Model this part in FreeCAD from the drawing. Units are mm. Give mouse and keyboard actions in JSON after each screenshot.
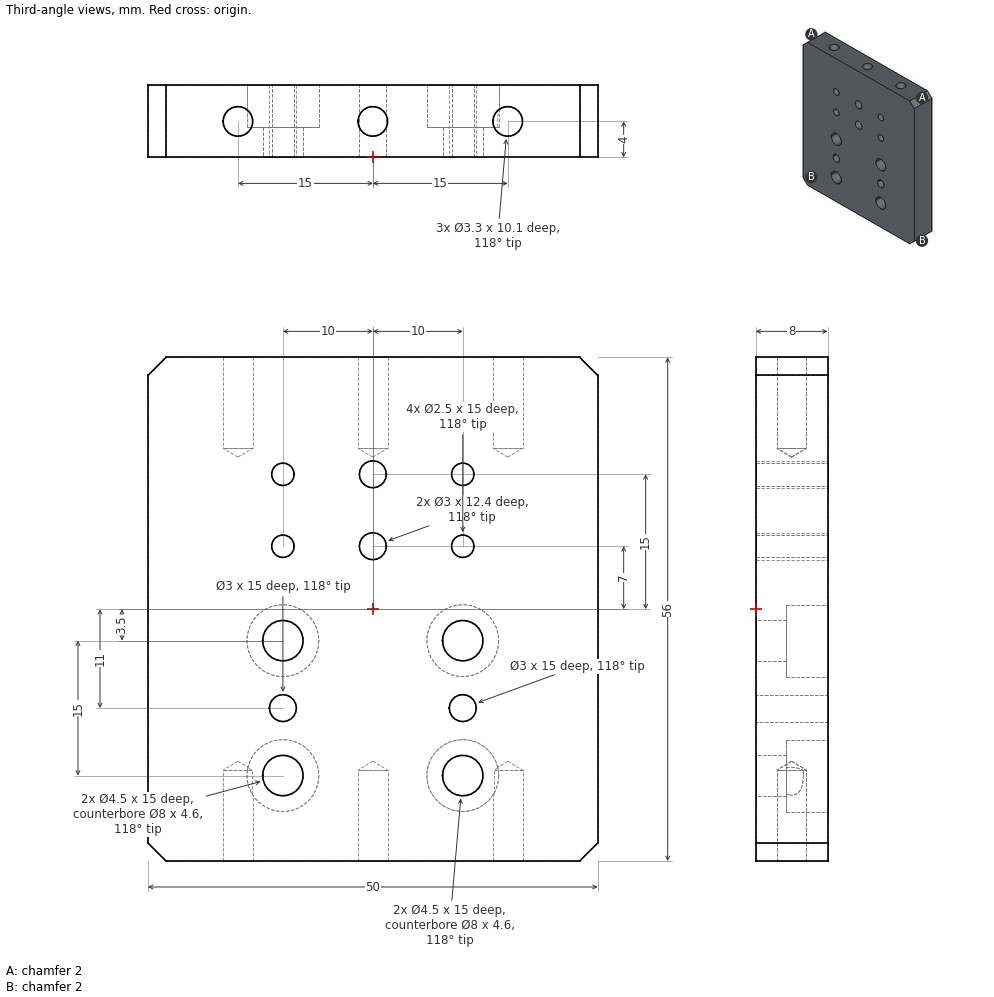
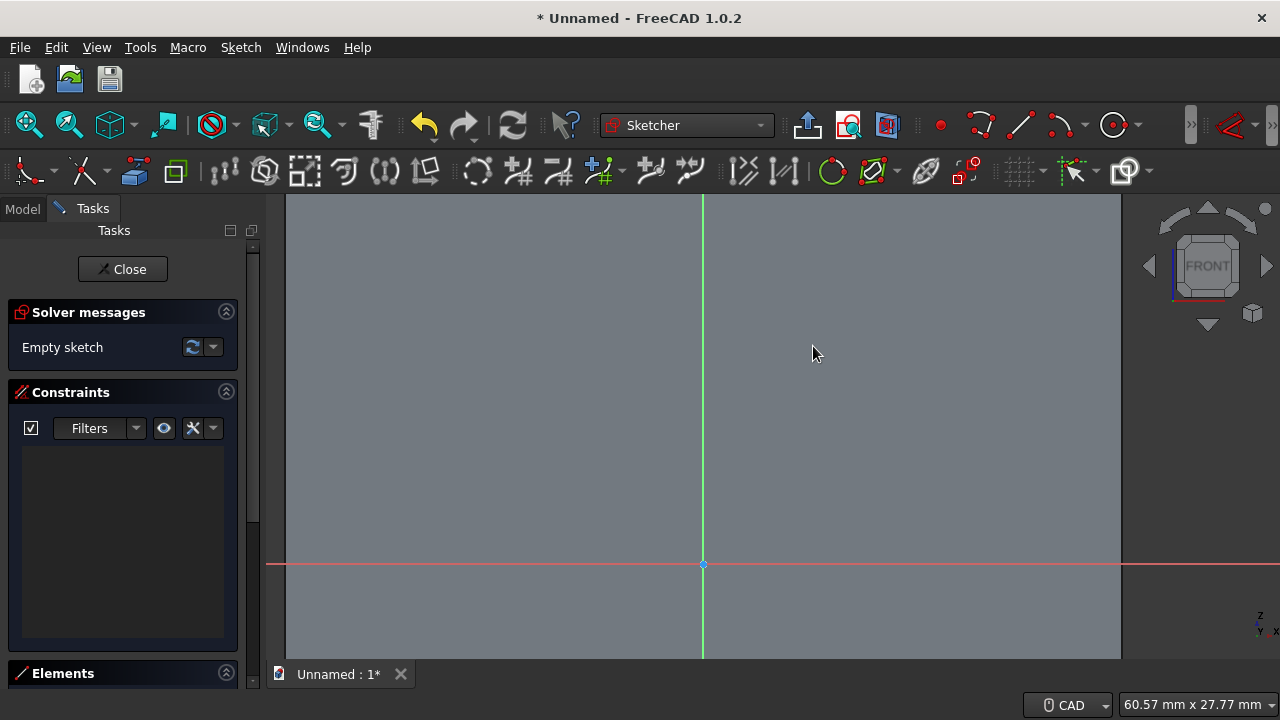
{"action": "left_click", "coordinate": [1114, 126]}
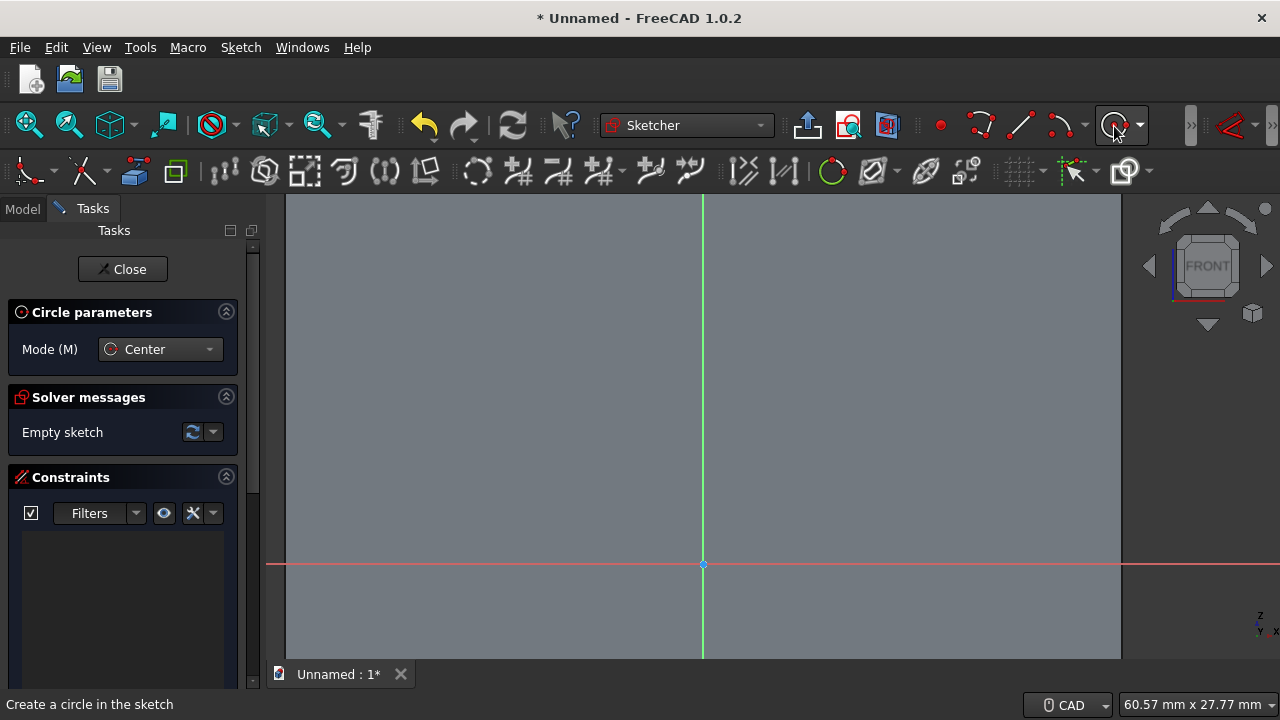
{"action": "left_click", "coordinate": [703, 447]}
{"action": "mouse_move", "coordinate": [721, 429]}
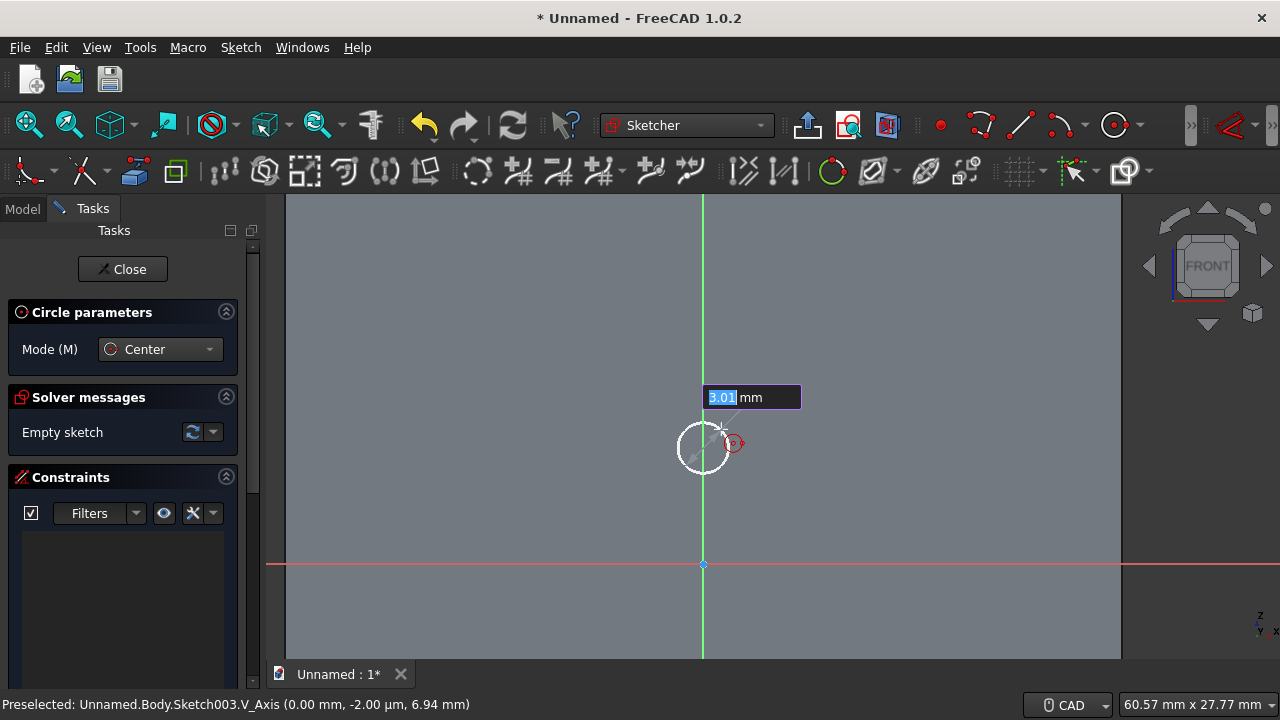
{"action": "type", "text": "3"}
{"action": "key", "text": "Return"}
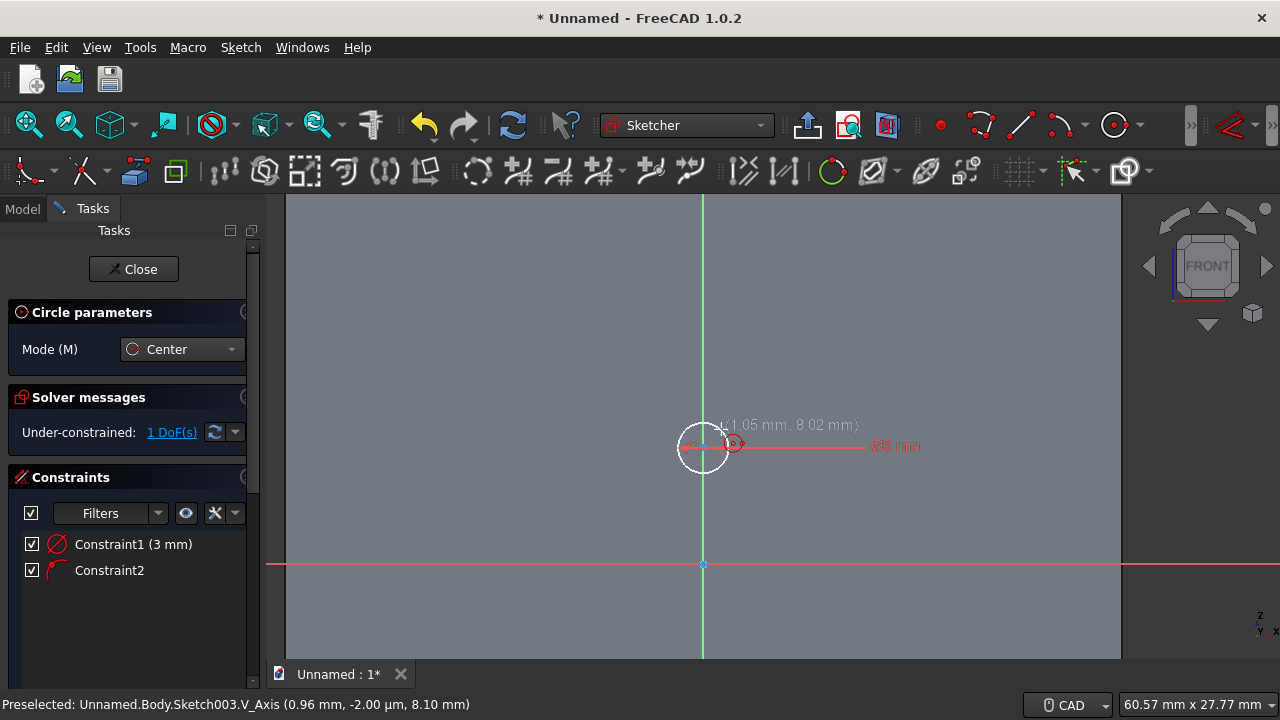
{"action": "left_click", "coordinate": [703, 313]}
{"action": "mouse_move", "coordinate": [721, 295]}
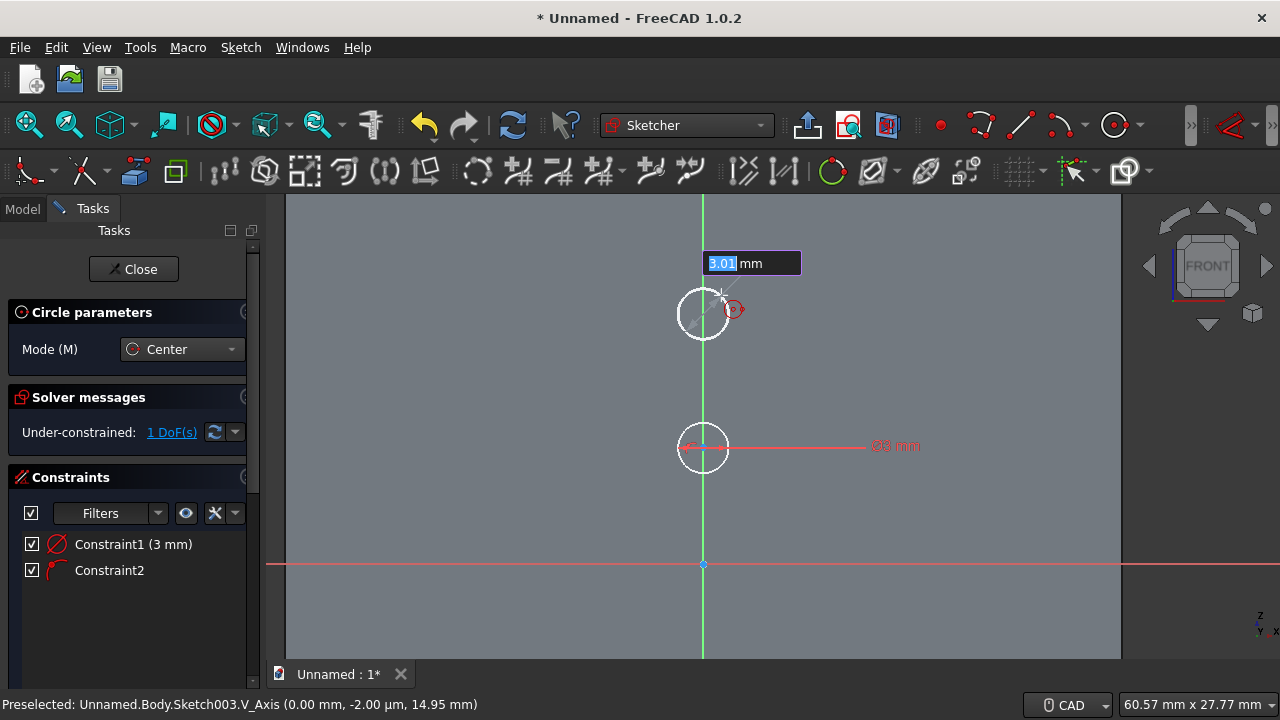
{"action": "type", "text": "3"}
{"action": "key", "text": "Return"}
{"action": "key", "text": "Escape"}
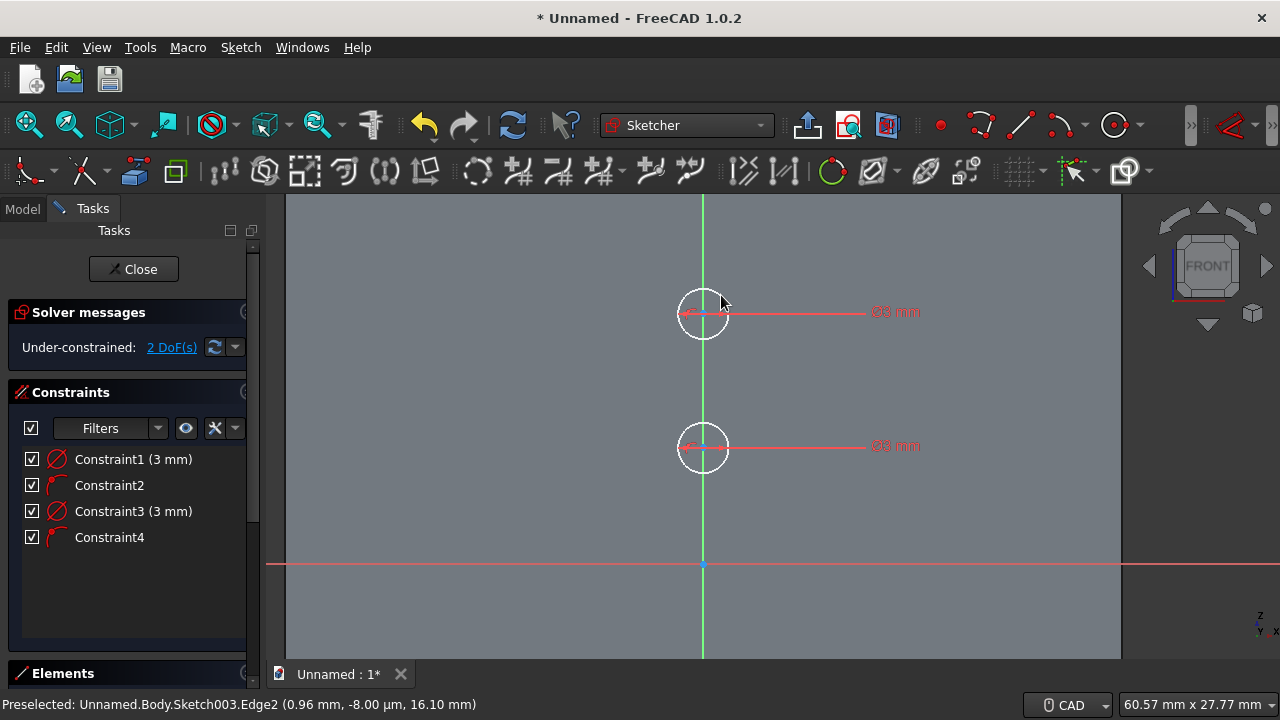
{"action": "left_click", "coordinate": [1230, 126]}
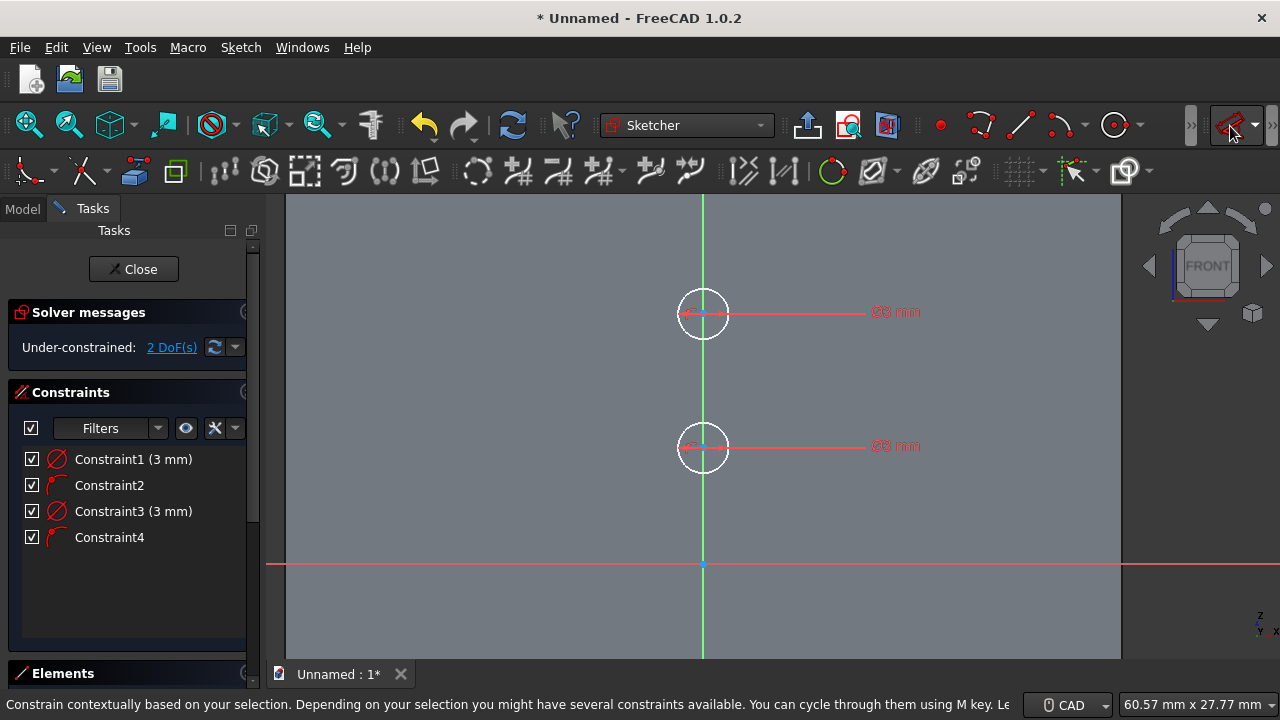
{"action": "left_click", "coordinate": [703, 448]}
{"action": "left_click", "coordinate": [737, 506]}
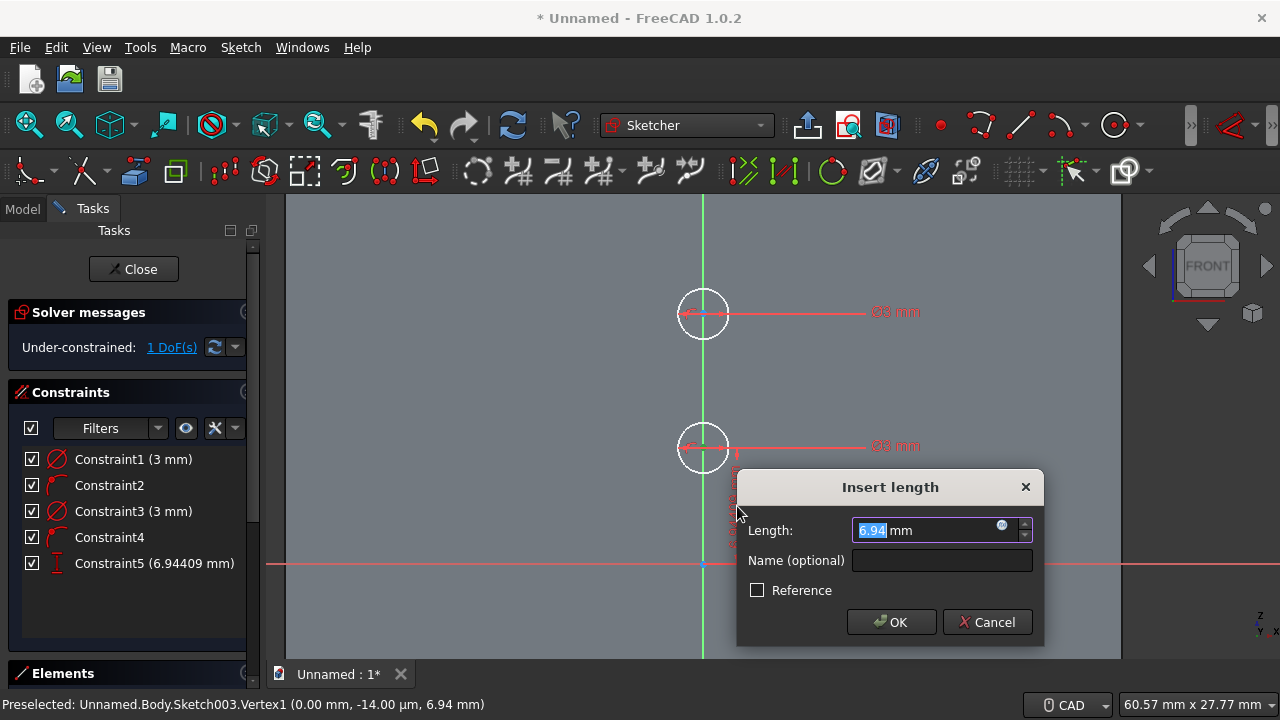
{"action": "type", "text": "7"}
{"action": "key", "text": "Return"}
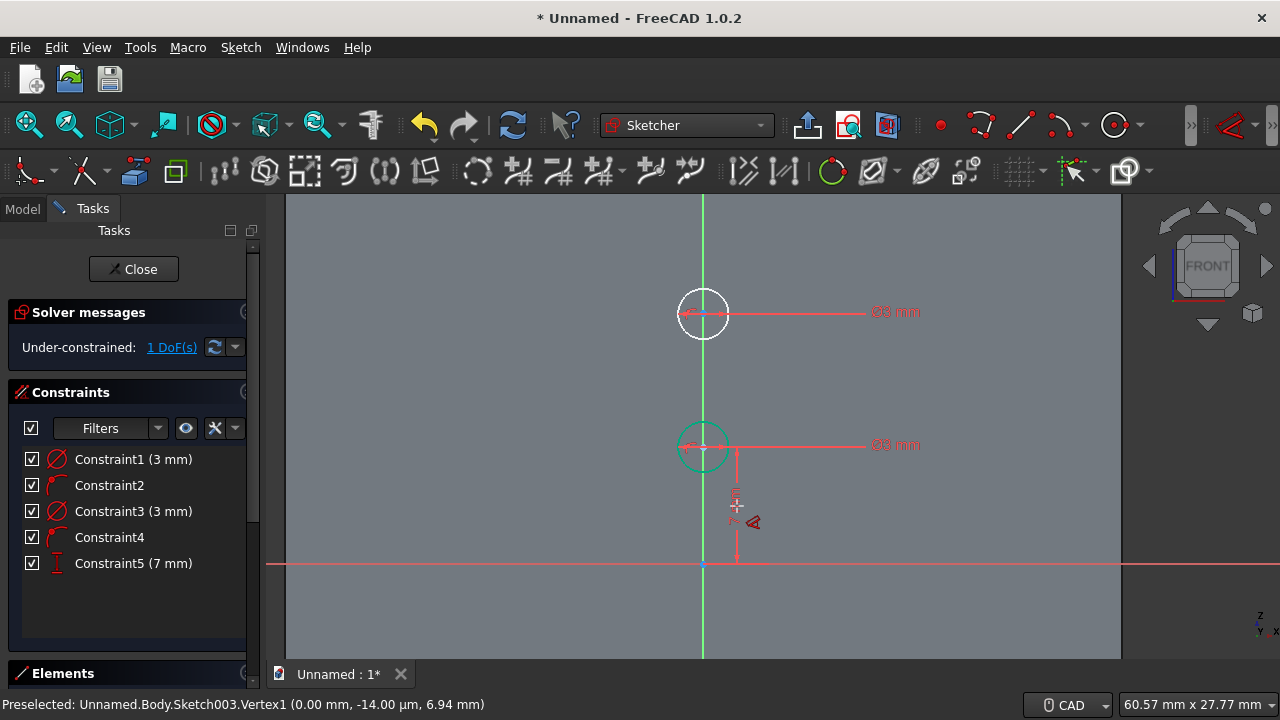
{"action": "left_click", "coordinate": [703, 314]}
{"action": "left_click", "coordinate": [737, 382]}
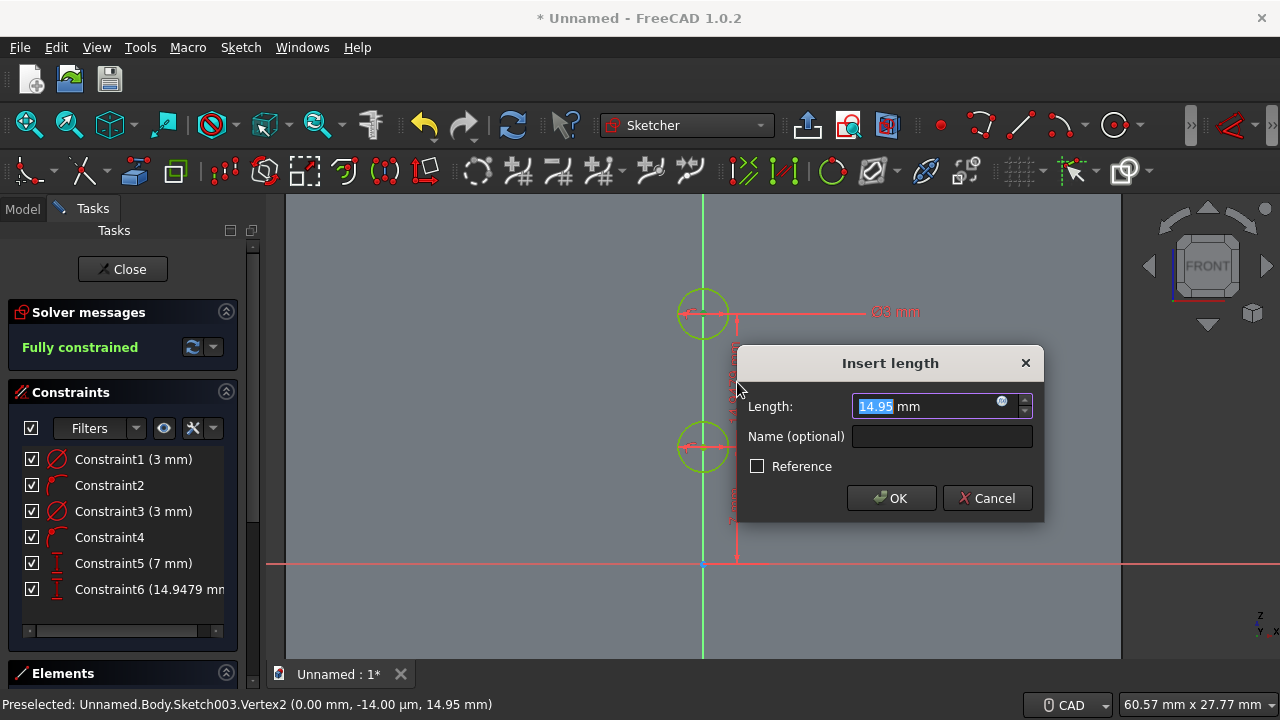
{"action": "type", "text": "15"}
{"action": "key", "text": "Return"}
{"action": "key", "text": "Escape"}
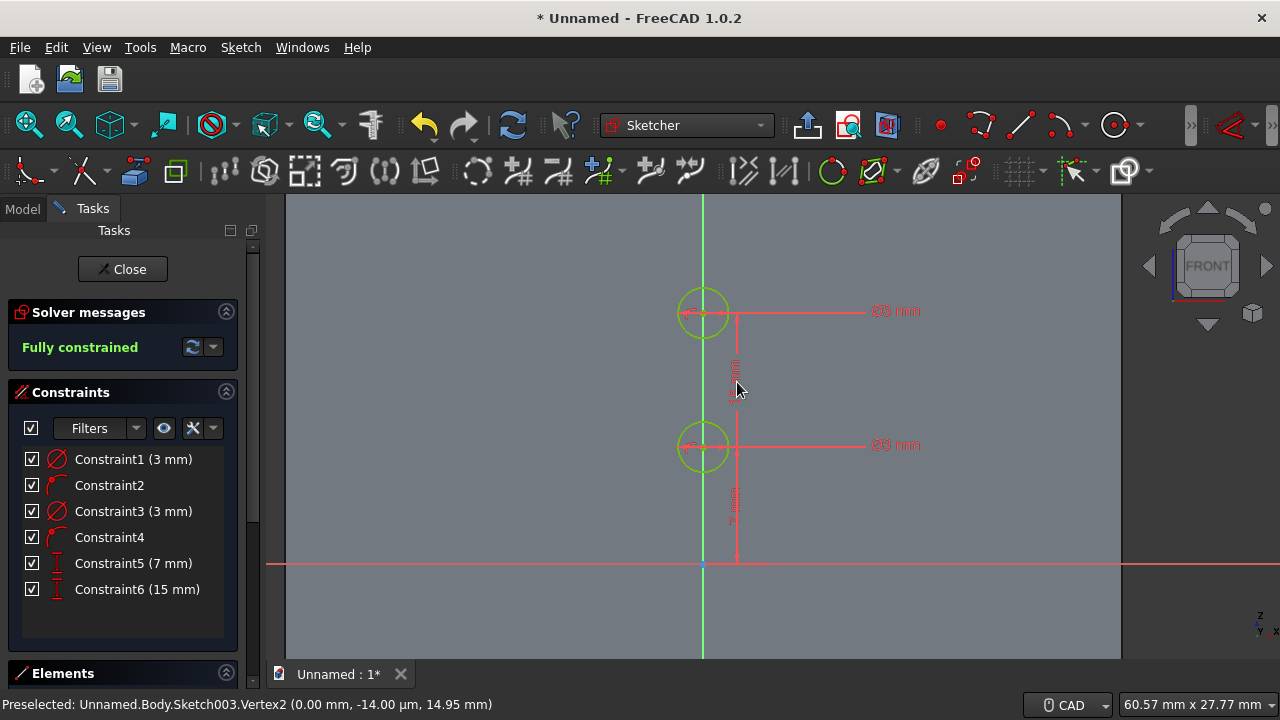
{"action": "left_click", "coordinate": [123, 269]}